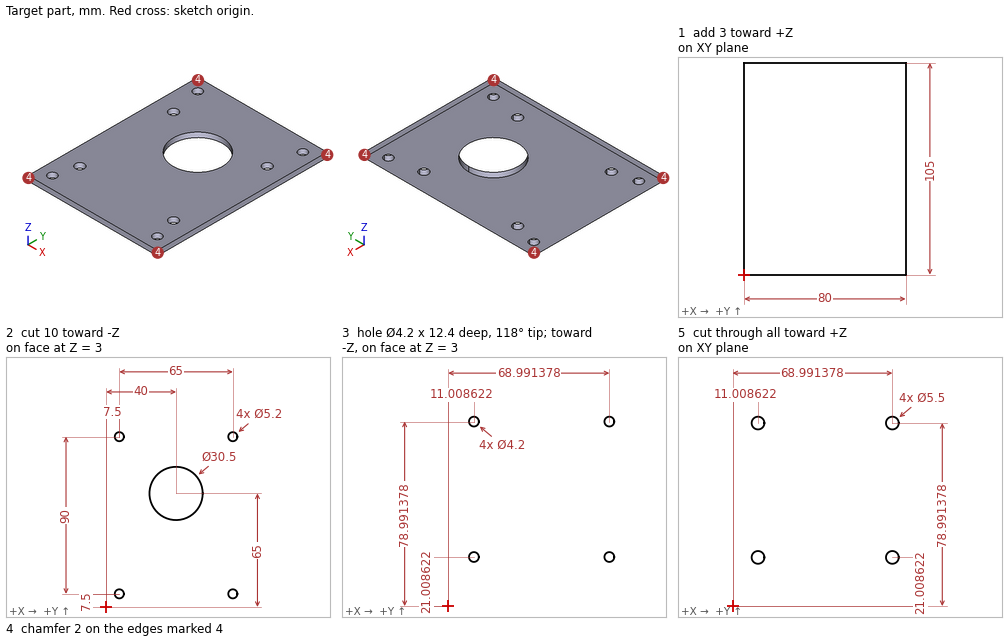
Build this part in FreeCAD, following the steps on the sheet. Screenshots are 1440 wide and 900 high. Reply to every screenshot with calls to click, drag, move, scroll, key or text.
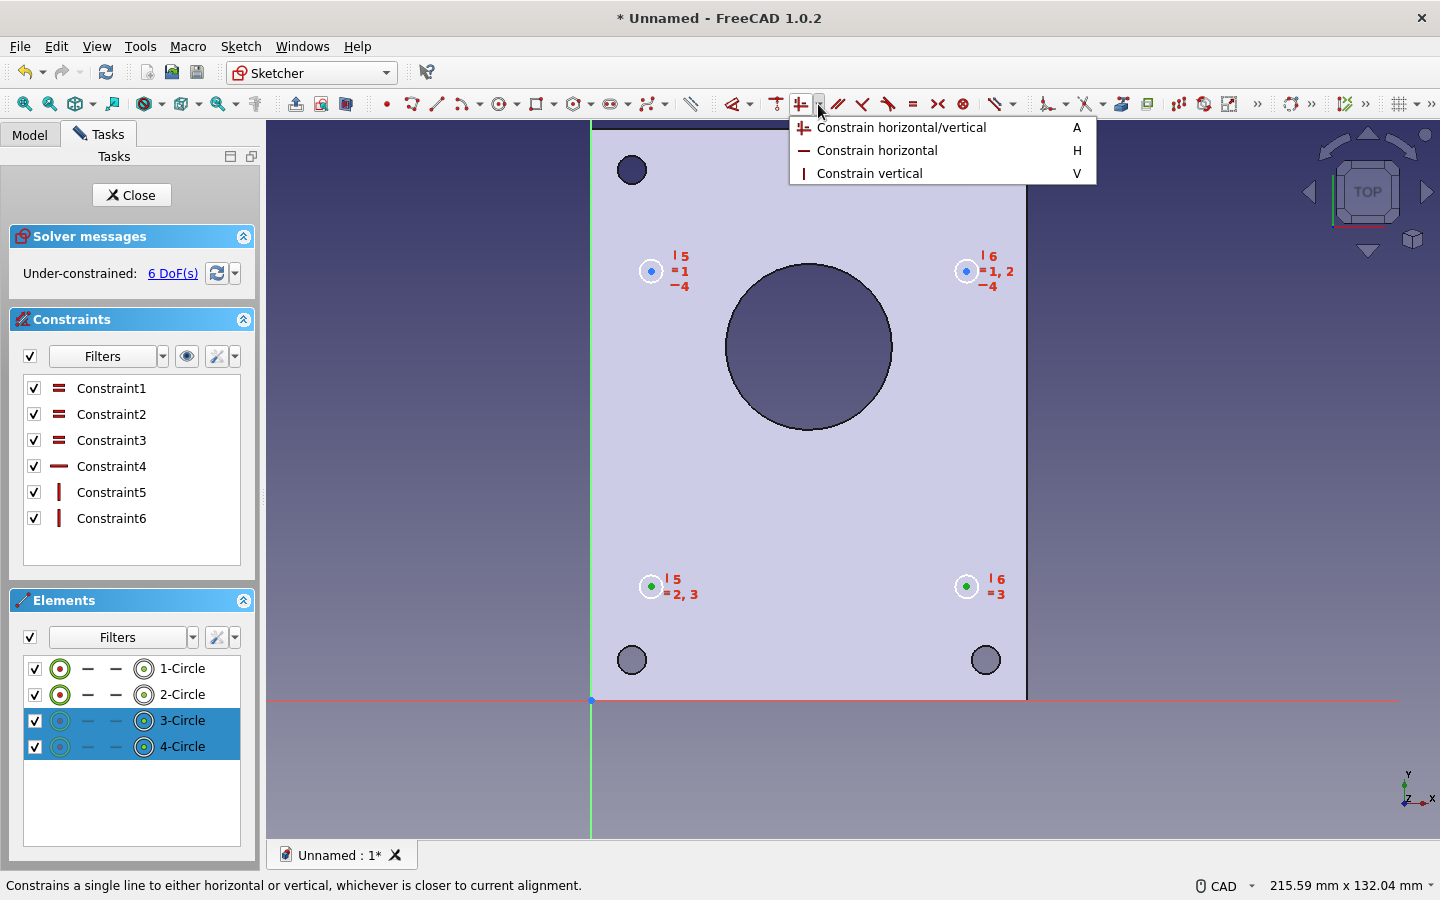
click(943, 150)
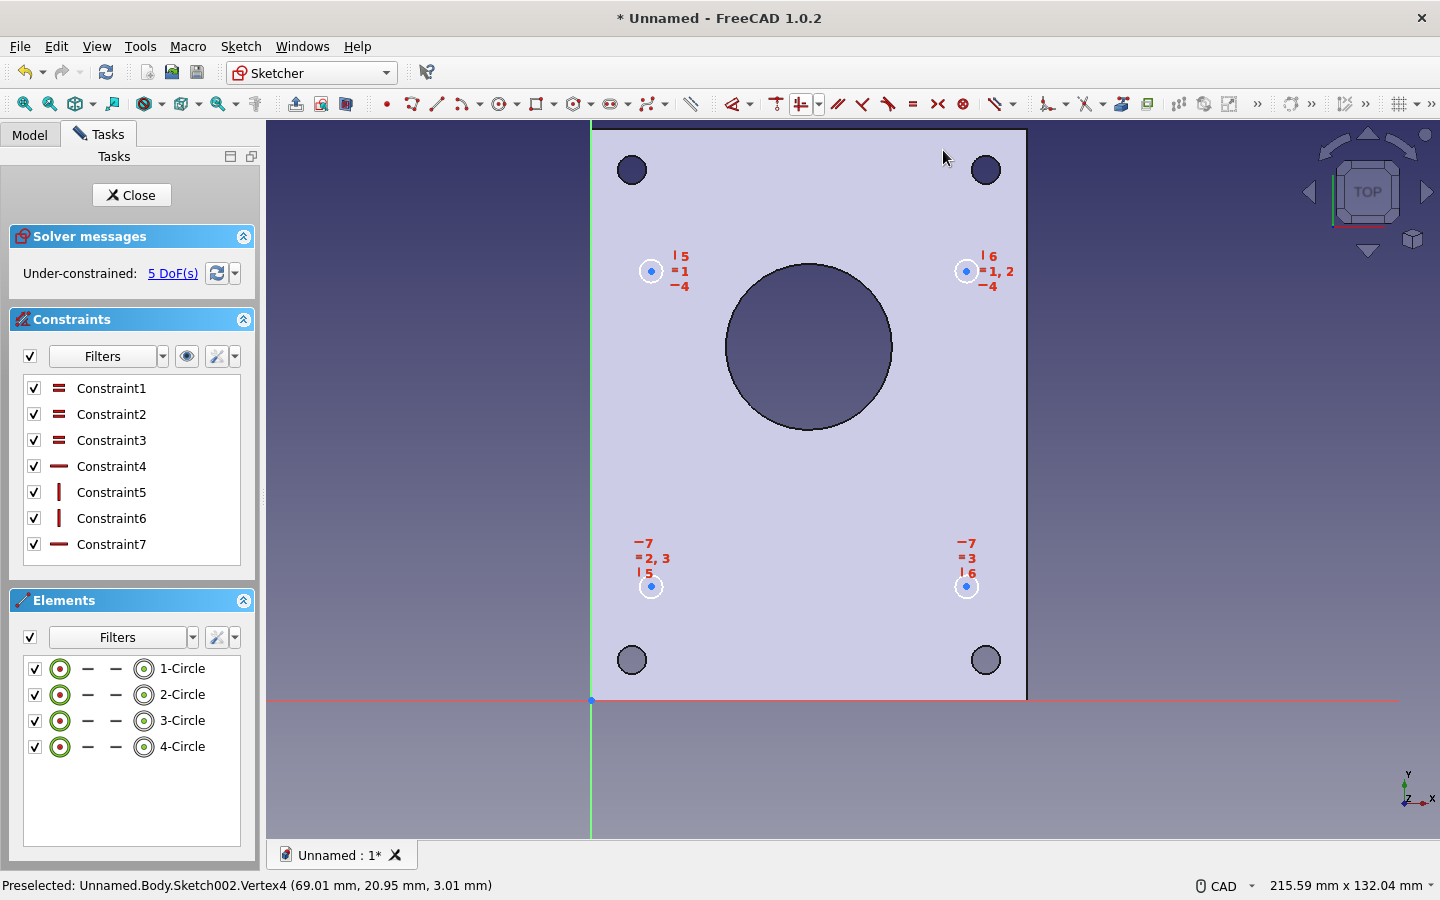
click(732, 104)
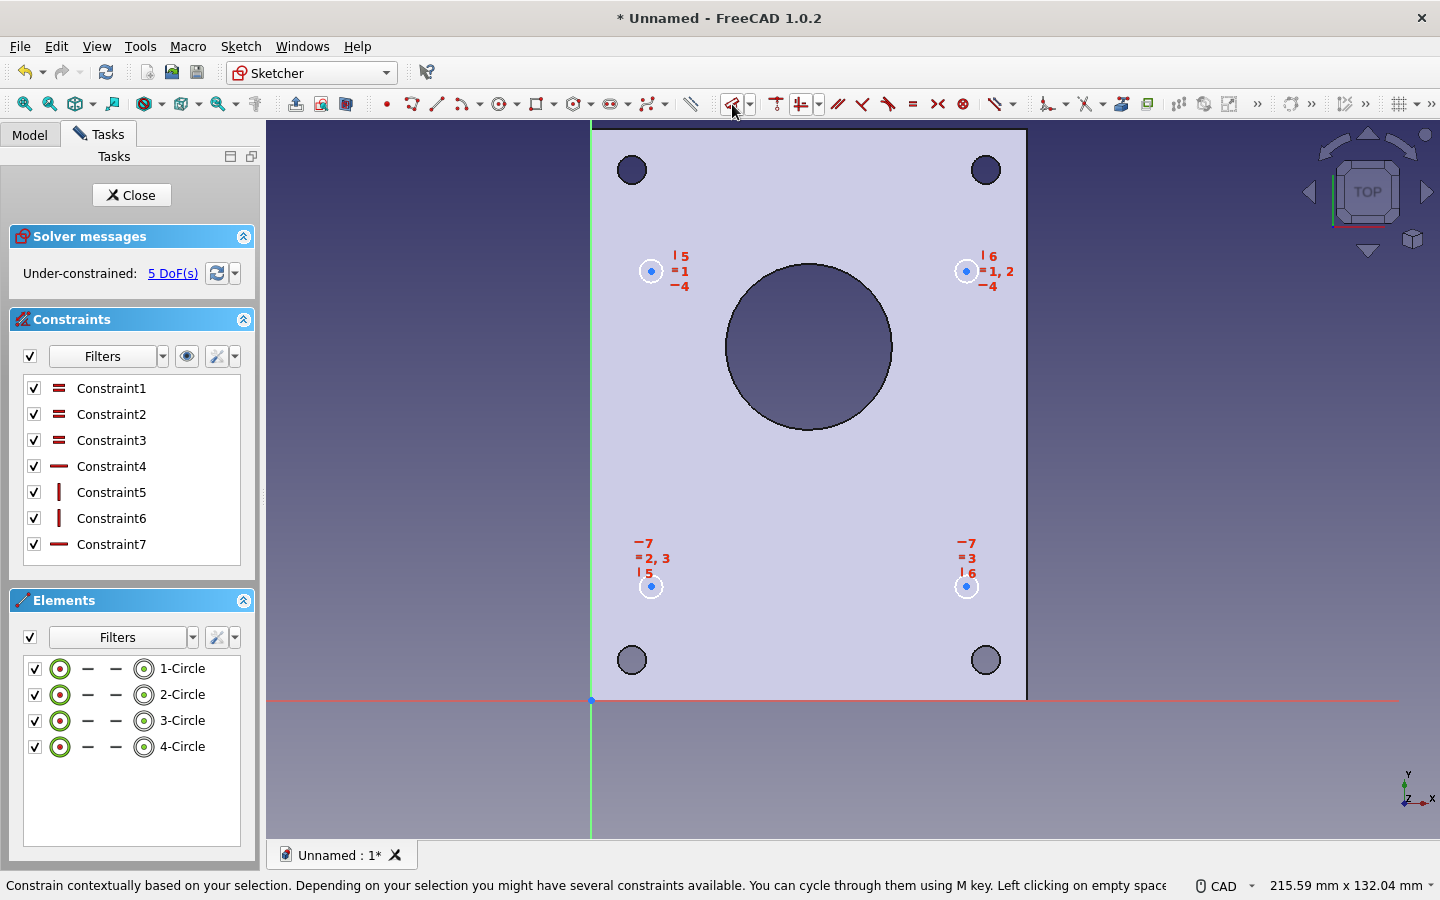
scroll(659, 263, up, 3)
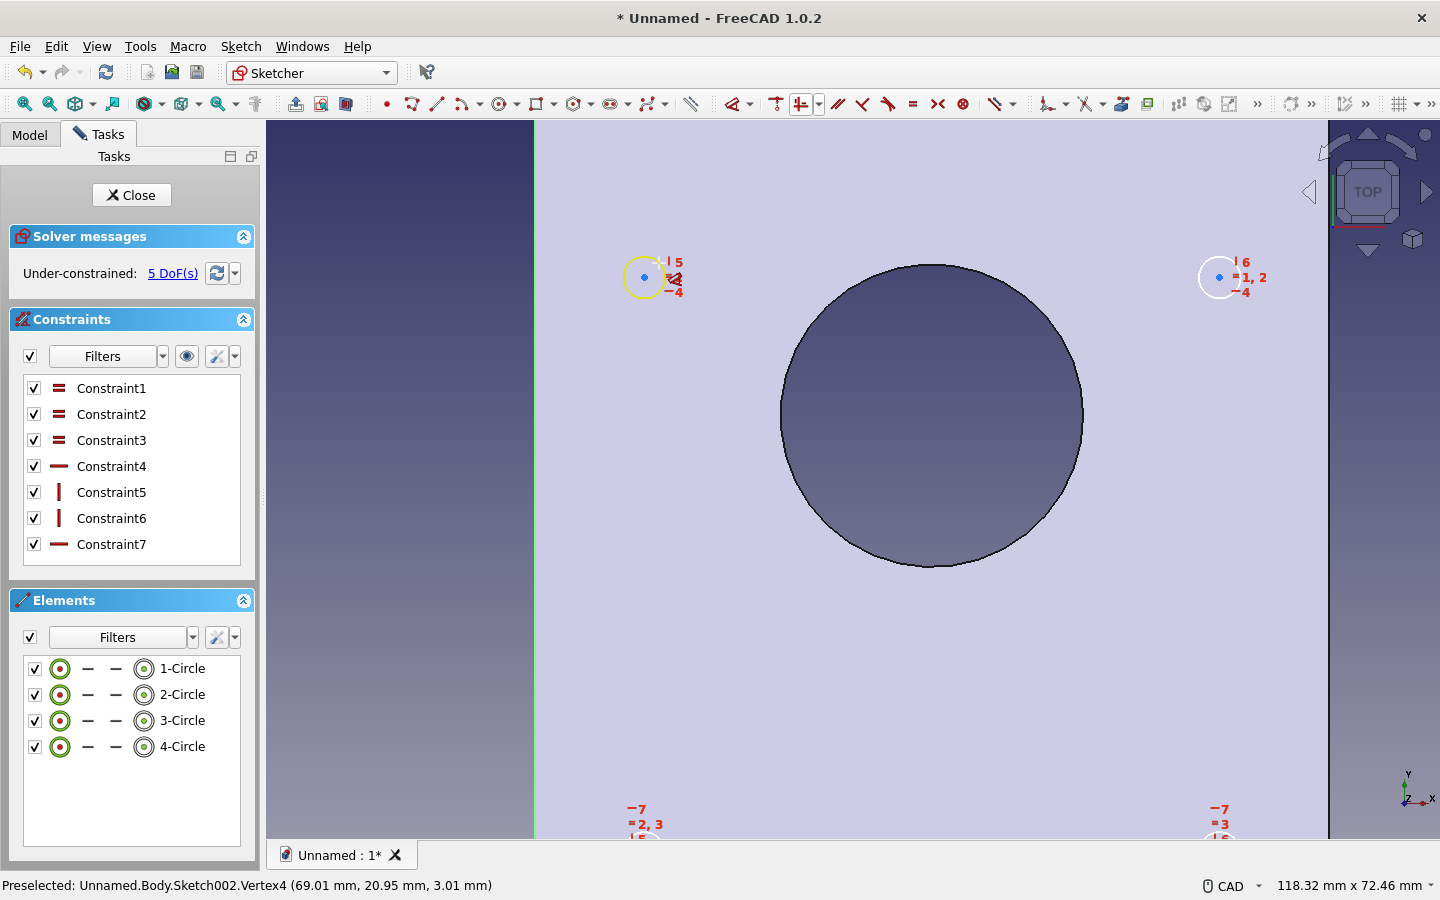
click(659, 263)
click(682, 240)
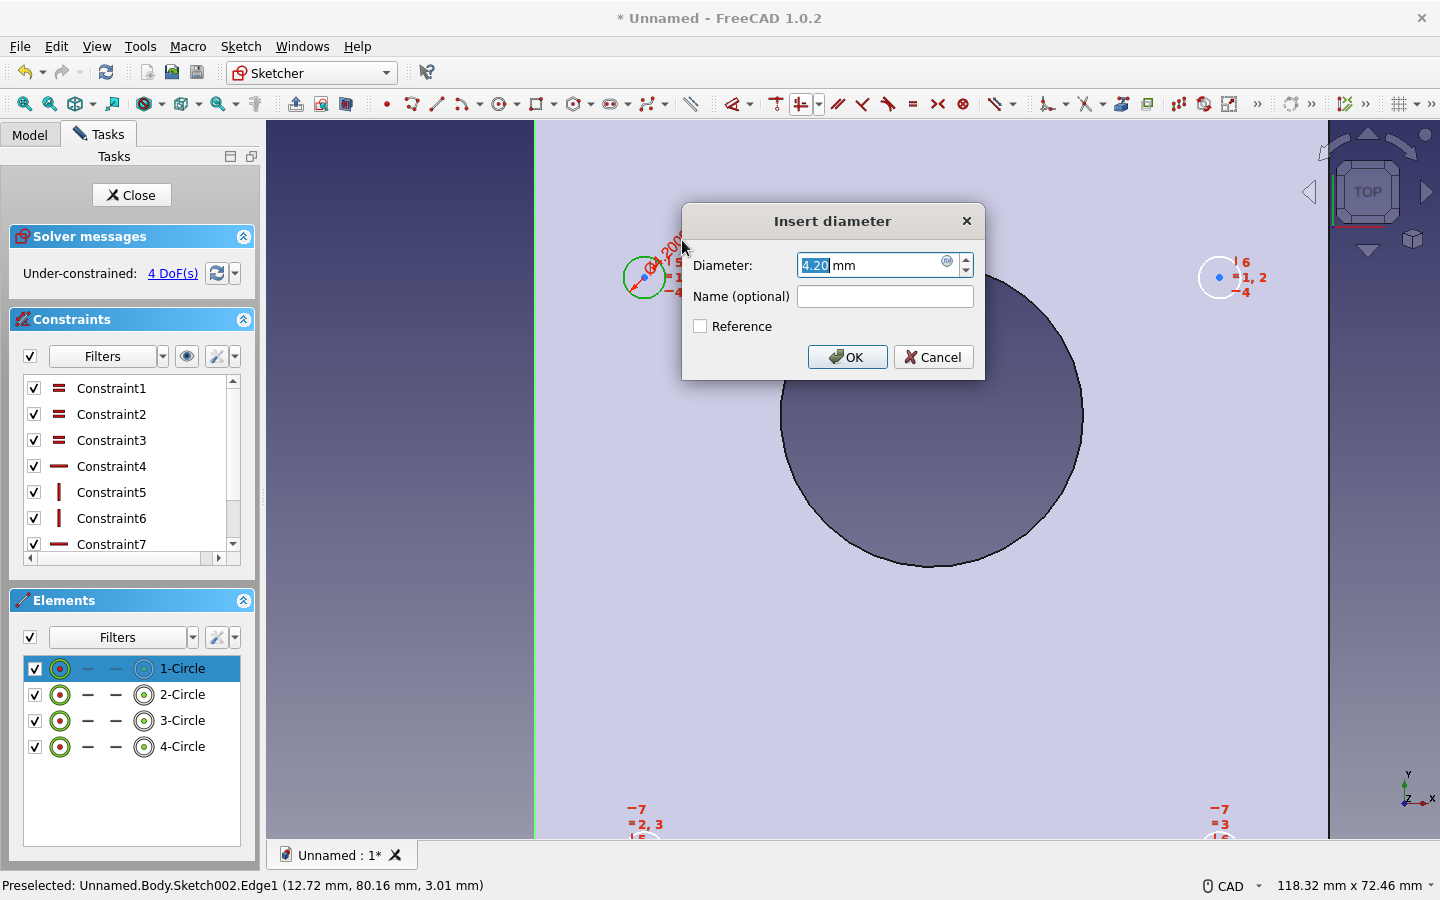
text(4.2)
key(Return)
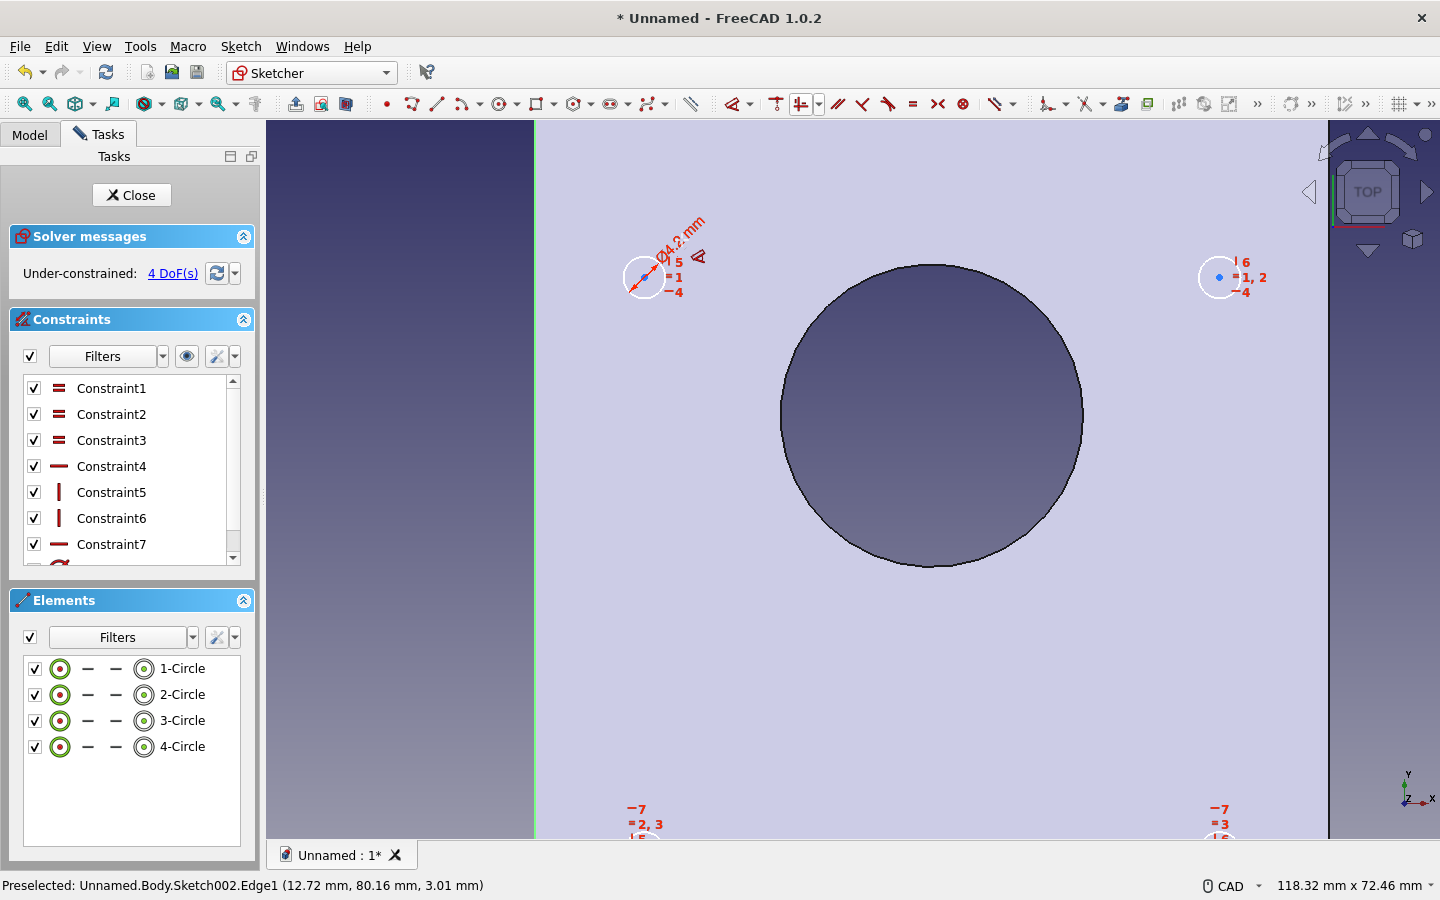
click(644, 278)
click(590, 244)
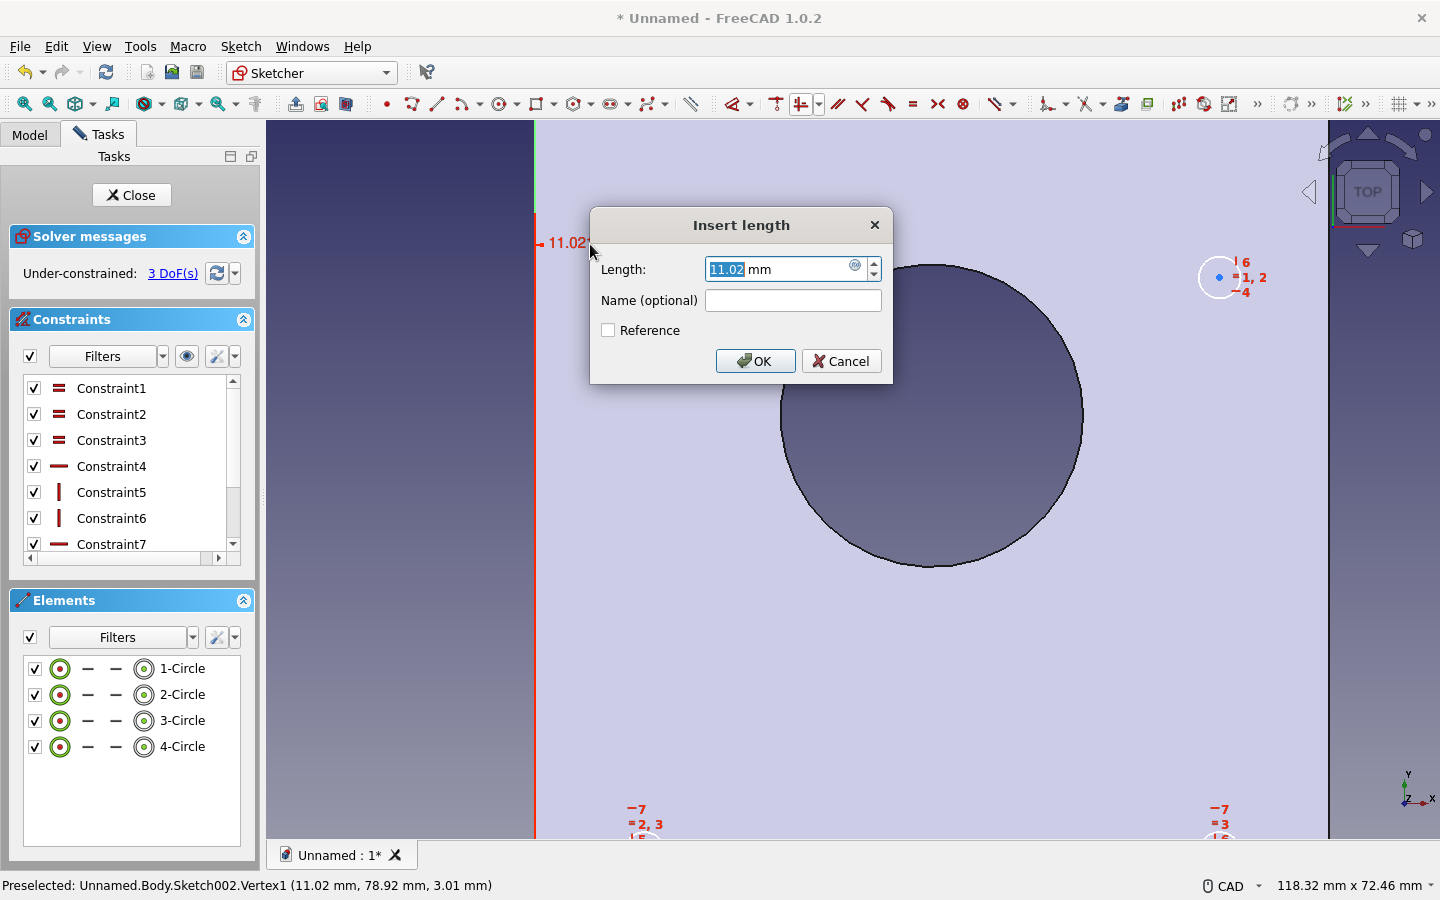
text(11.008622)
key(Return)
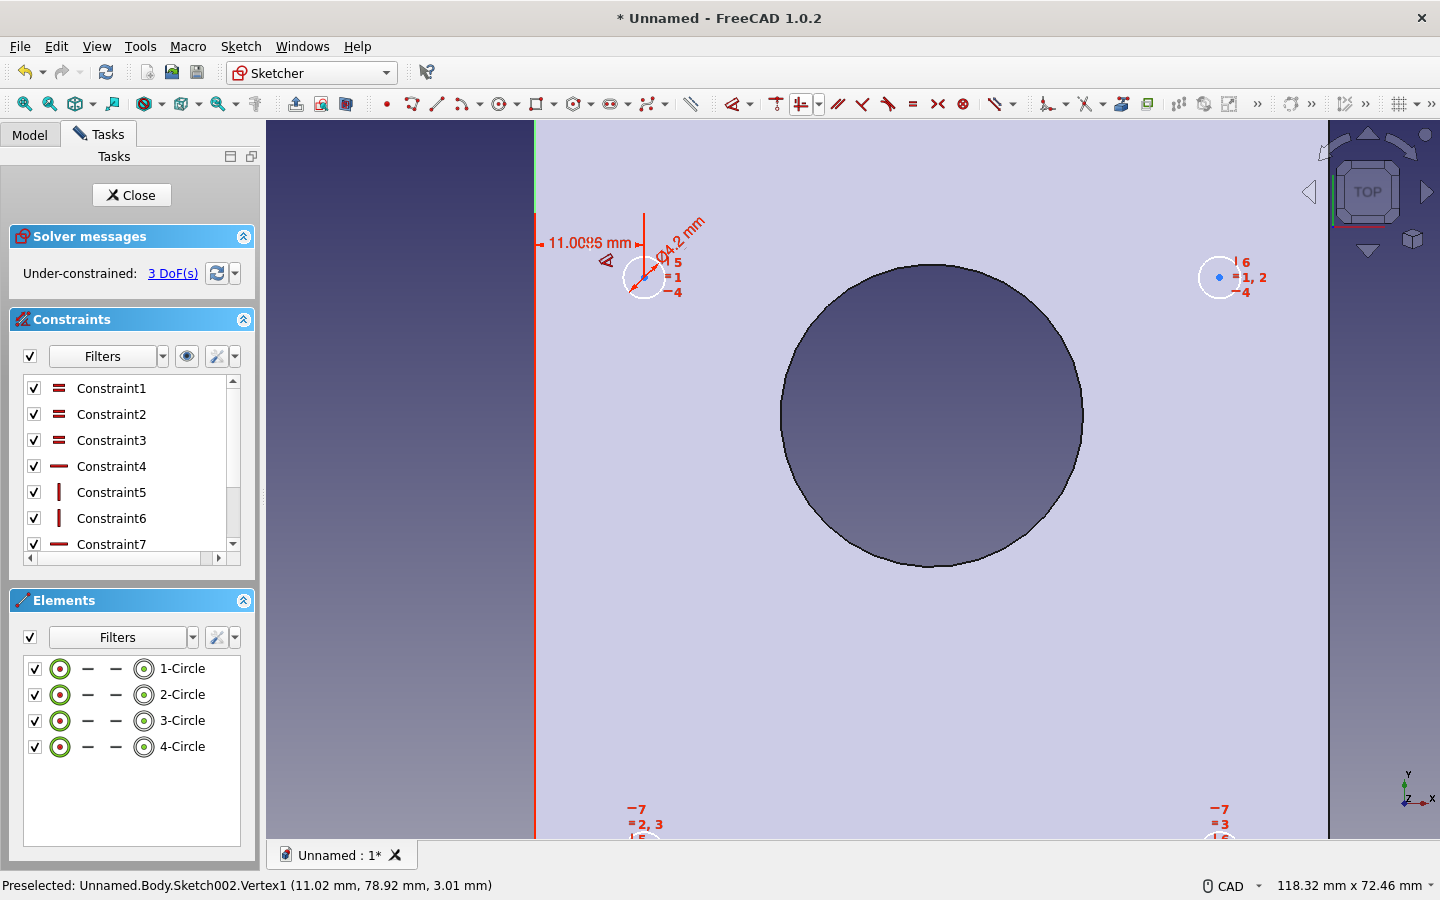
click(644, 278)
click(501, 544)